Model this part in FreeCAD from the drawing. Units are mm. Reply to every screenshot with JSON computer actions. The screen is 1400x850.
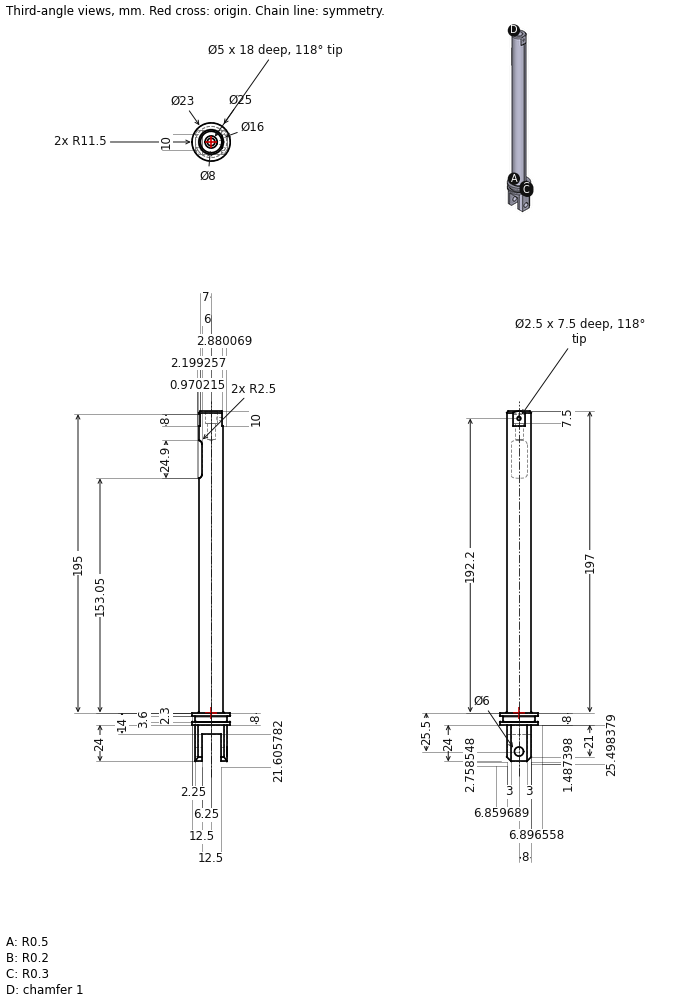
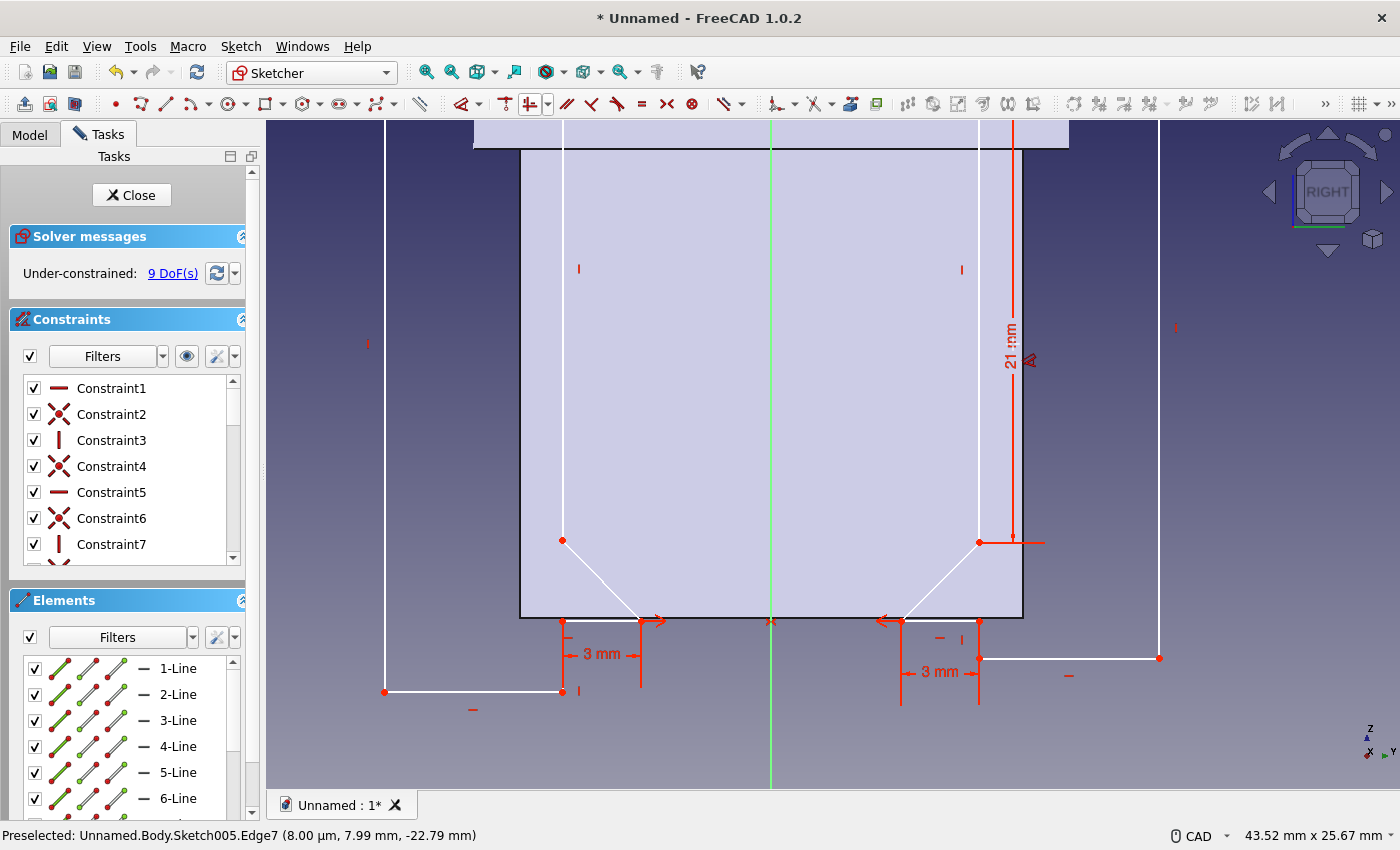
{"action": "left_click", "coordinate": [563, 159]}
{"action": "left_click", "coordinate": [529, 344]}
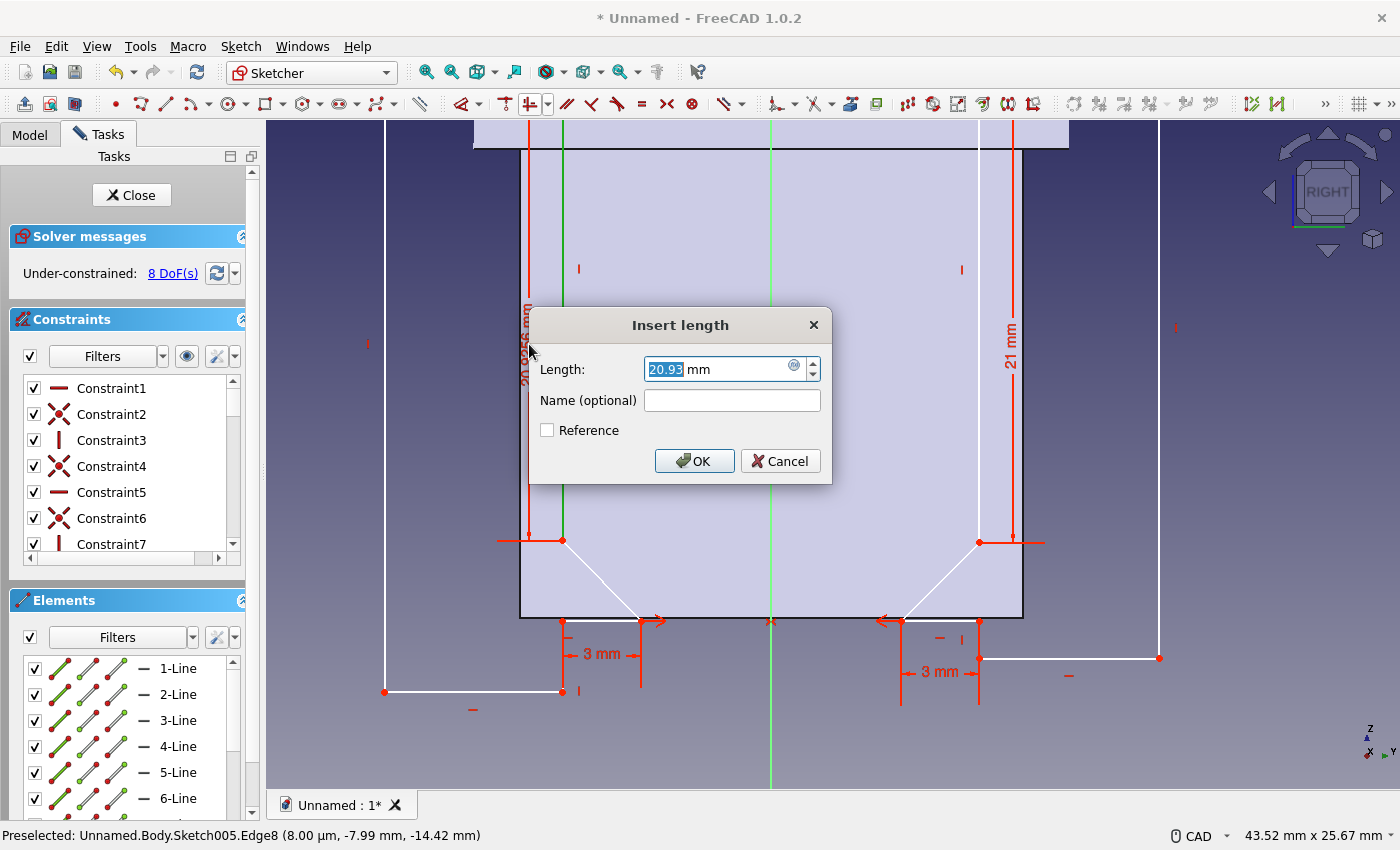
{"action": "type", "text": "21"}
{"action": "key", "text": "Return"}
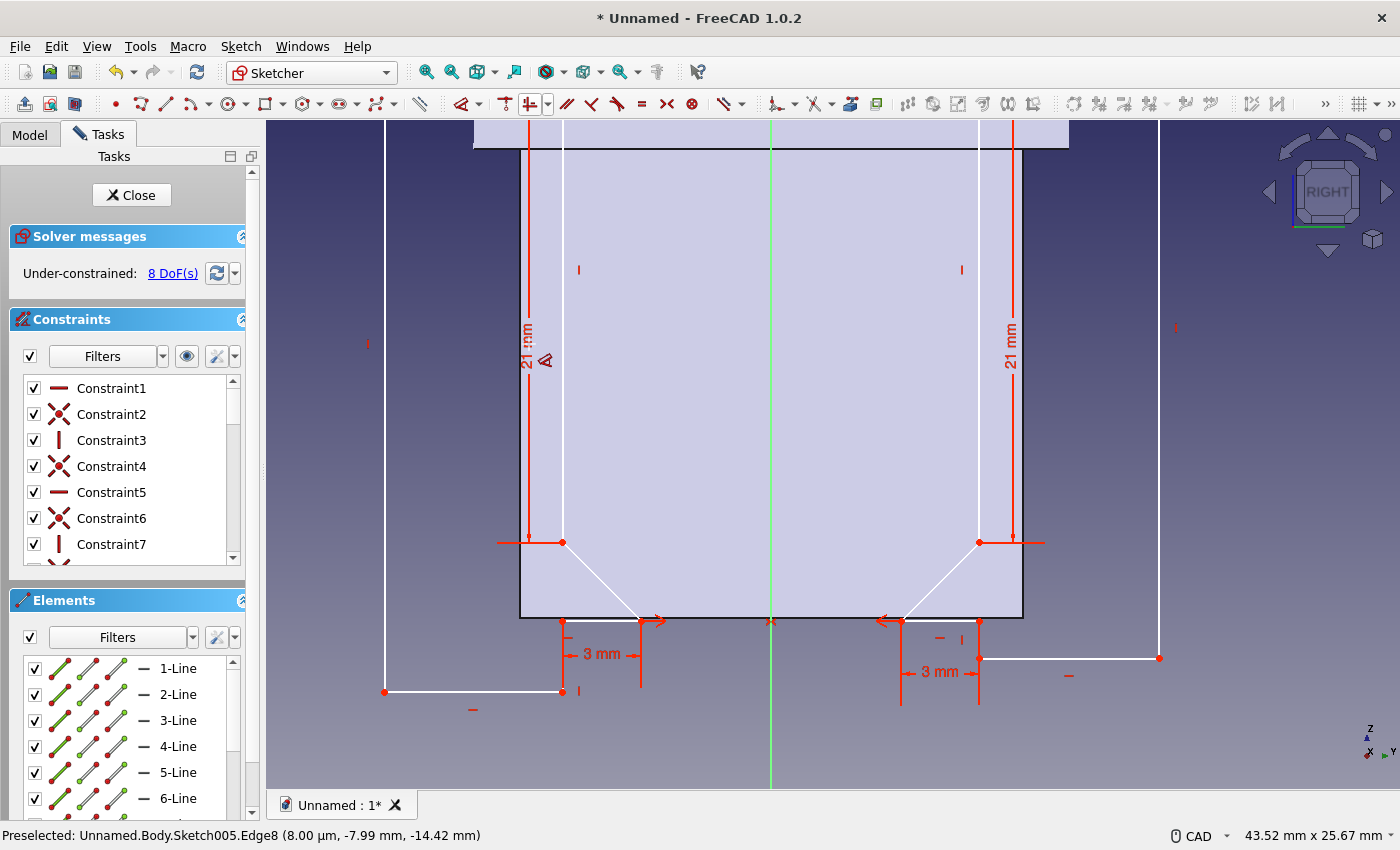
{"action": "scroll", "coordinate": [759, 632], "scroll_direction": "down", "scroll_amount": 4}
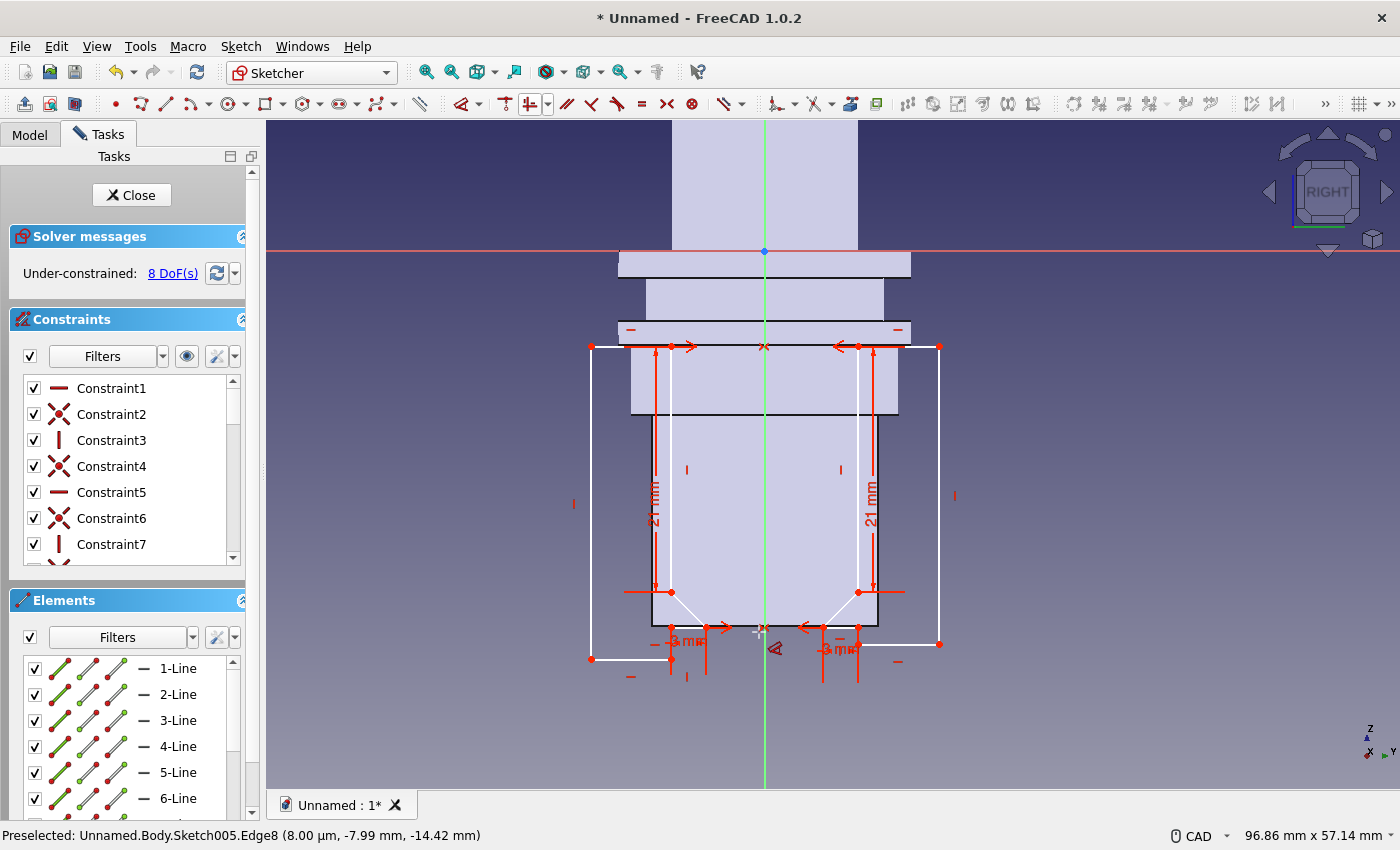
{"action": "left_click", "coordinate": [858, 347]}
{"action": "left_click", "coordinate": [811, 217]}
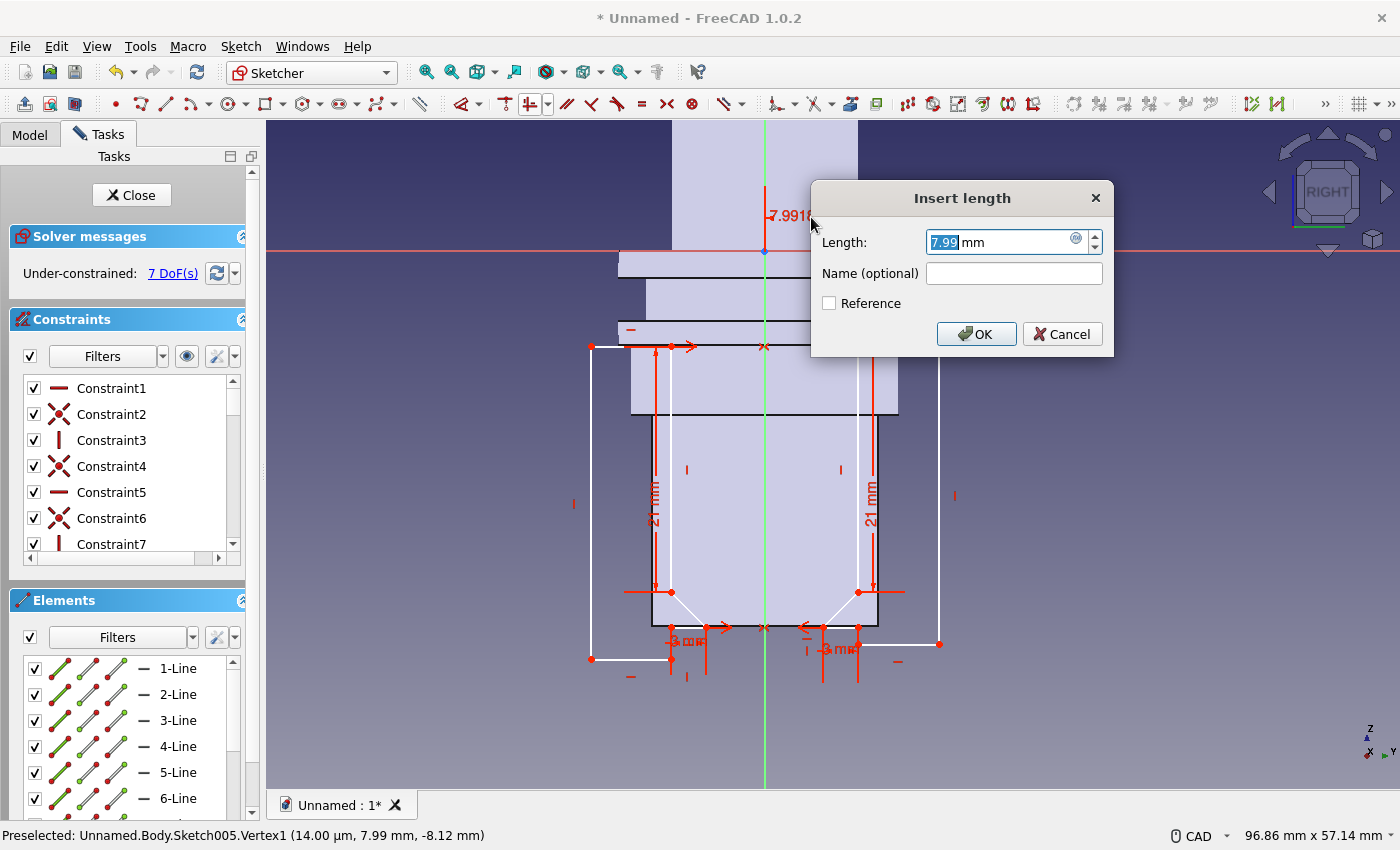
{"action": "type", "text": "8"}
{"action": "key", "text": "Return"}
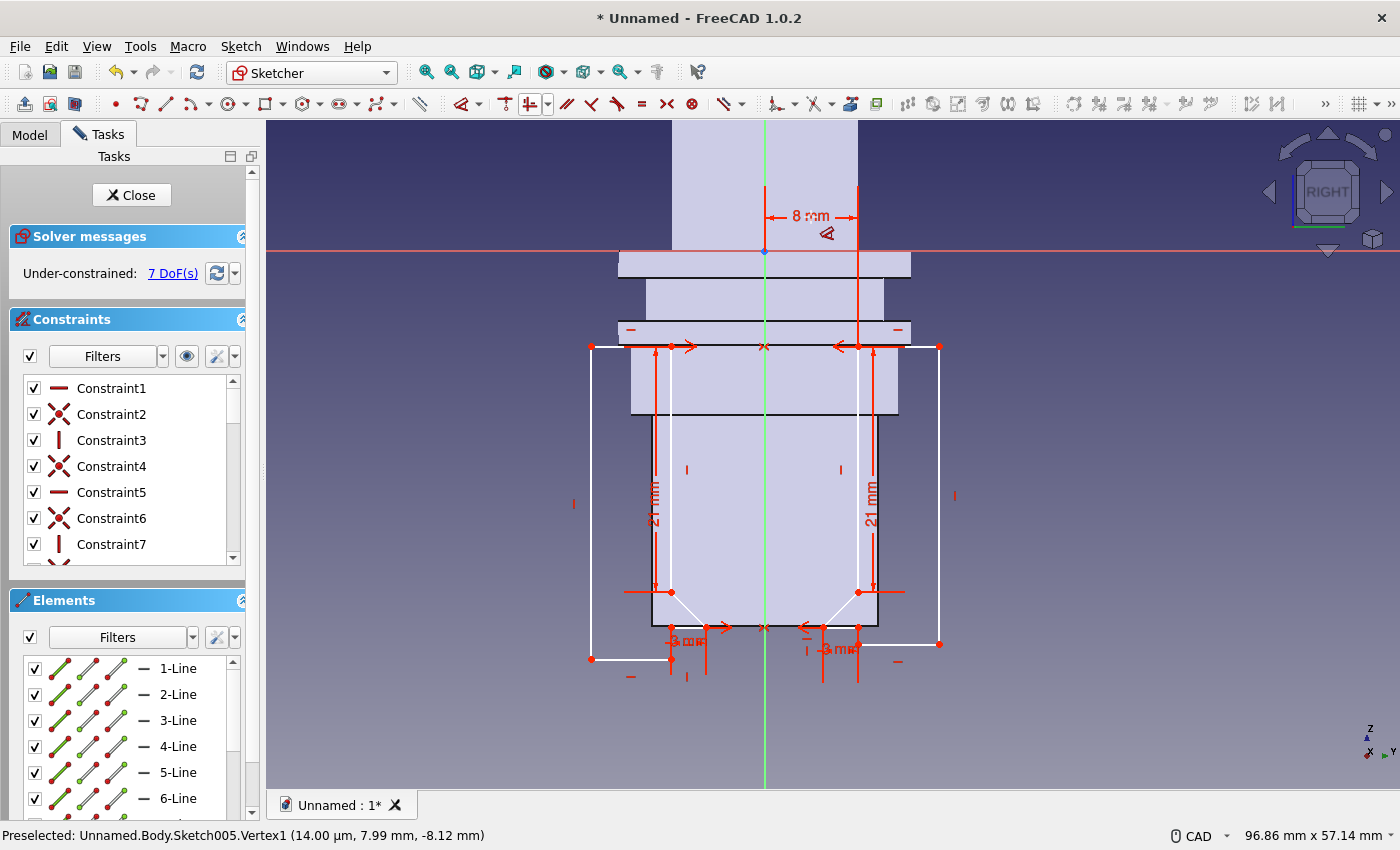
{"action": "left_click", "coordinate": [858, 347]}
{"action": "left_click", "coordinate": [892, 299]}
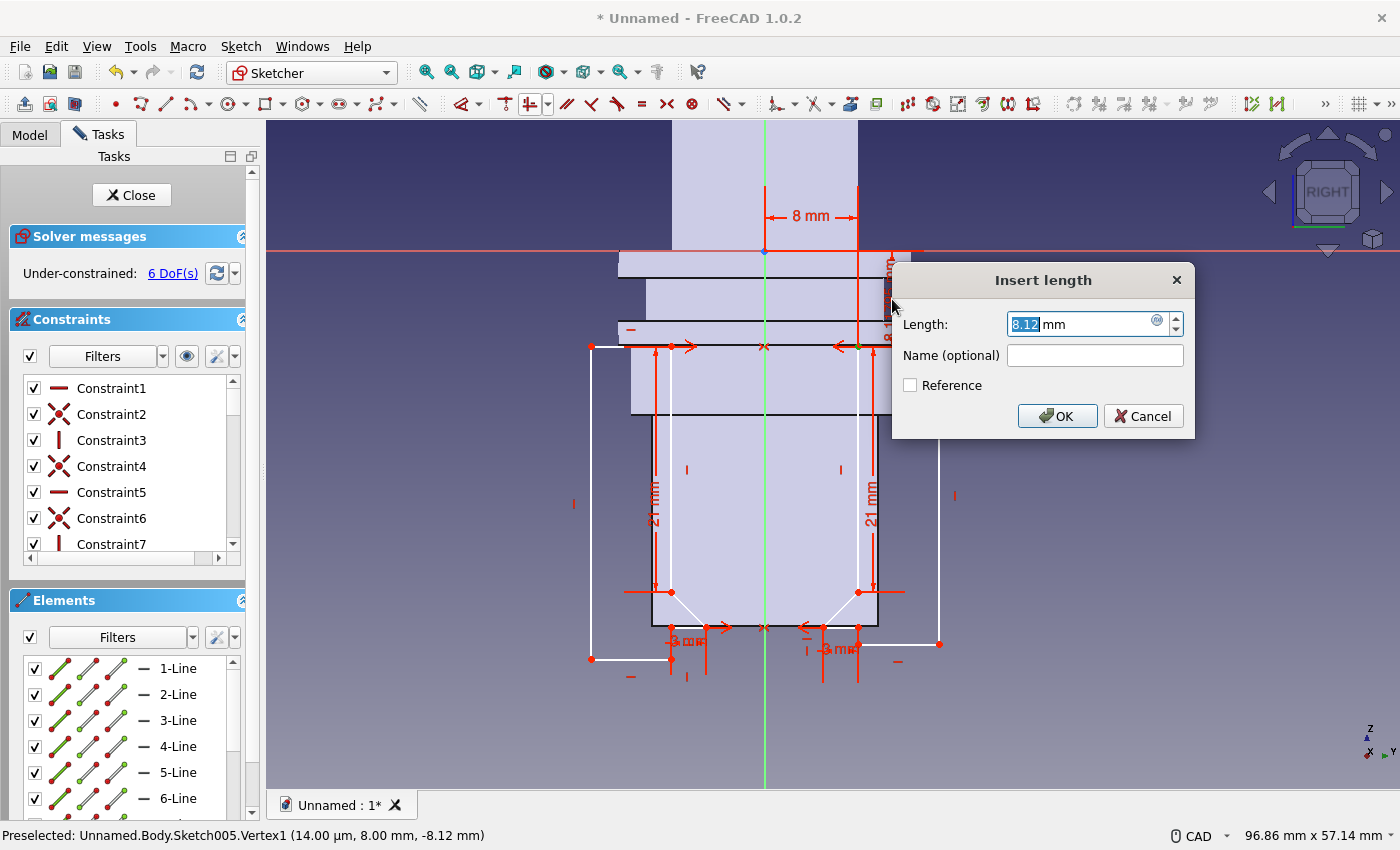
{"action": "type", "text": "8"}
{"action": "key", "text": "Return"}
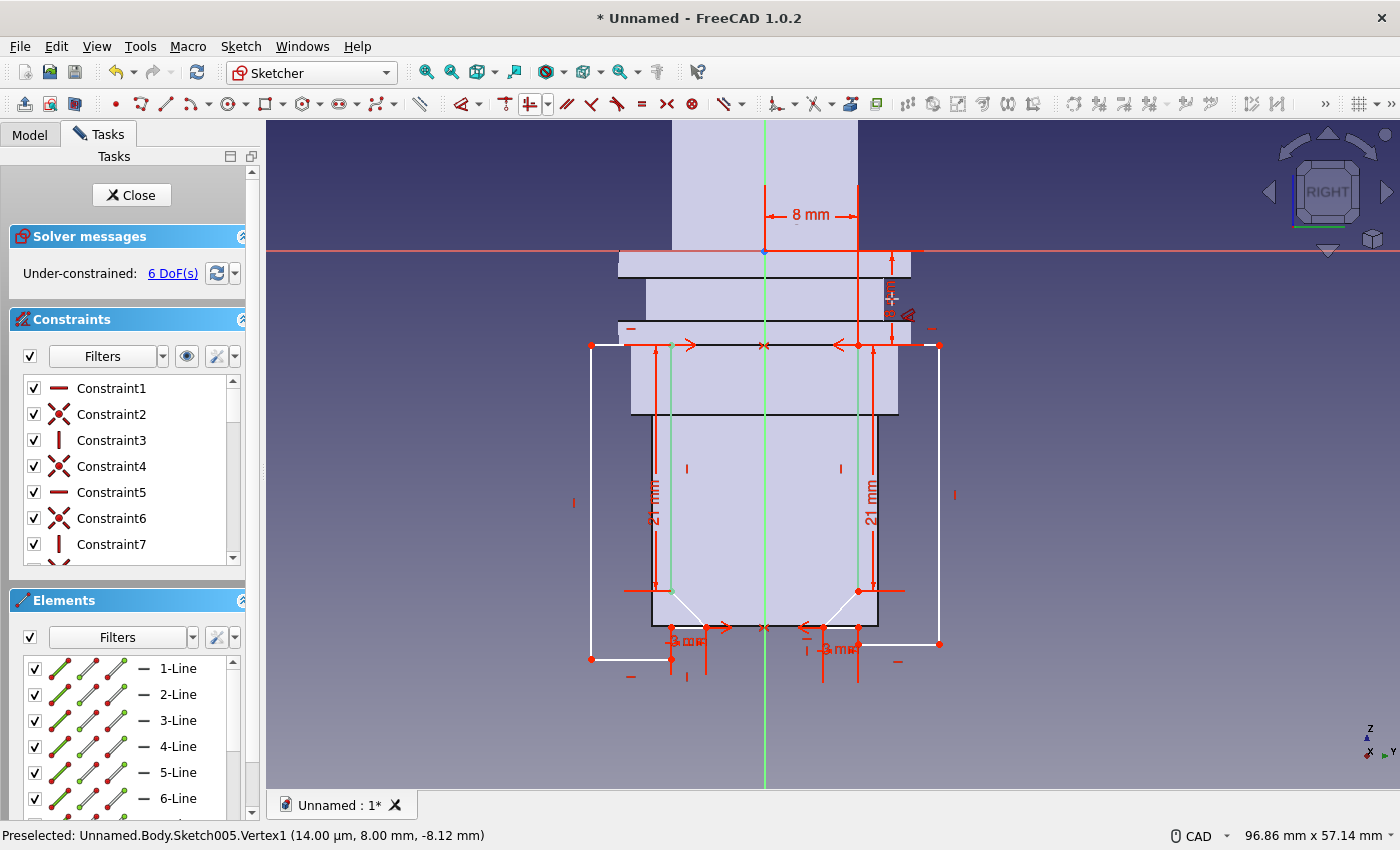
{"action": "left_click", "coordinate": [858, 645]}
{"action": "left_click", "coordinate": [811, 679]}